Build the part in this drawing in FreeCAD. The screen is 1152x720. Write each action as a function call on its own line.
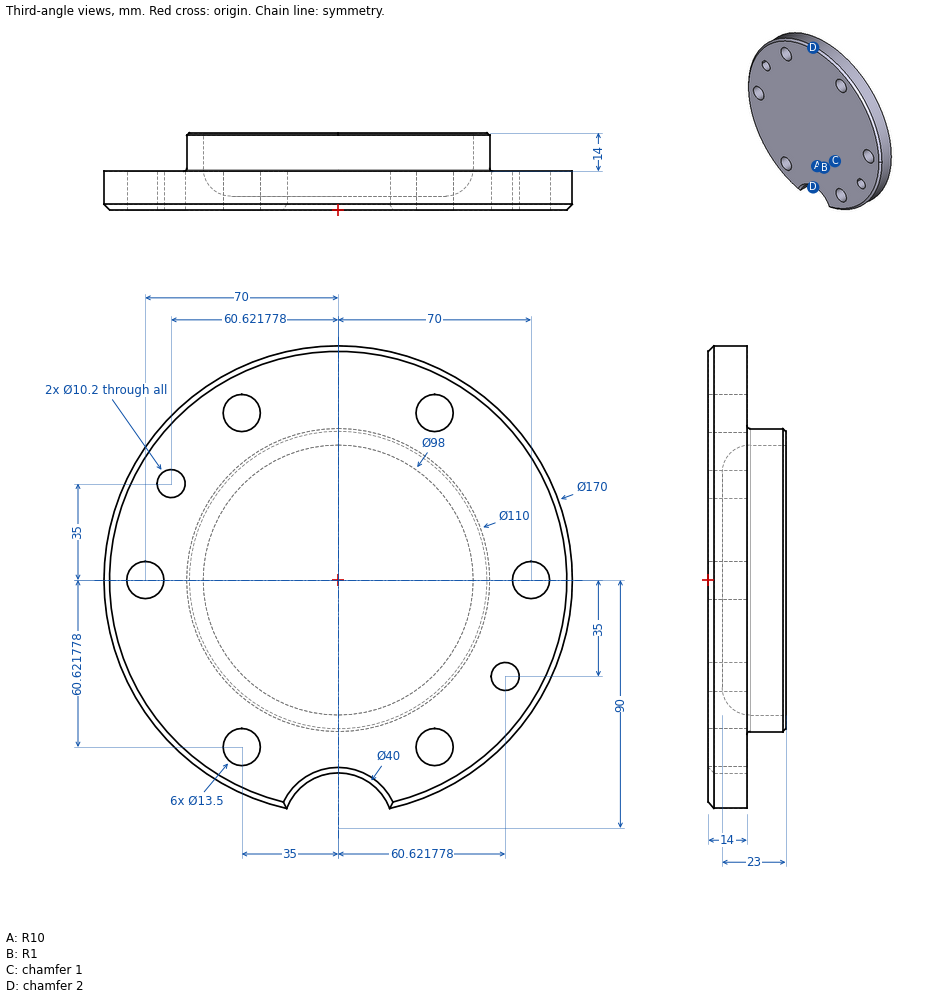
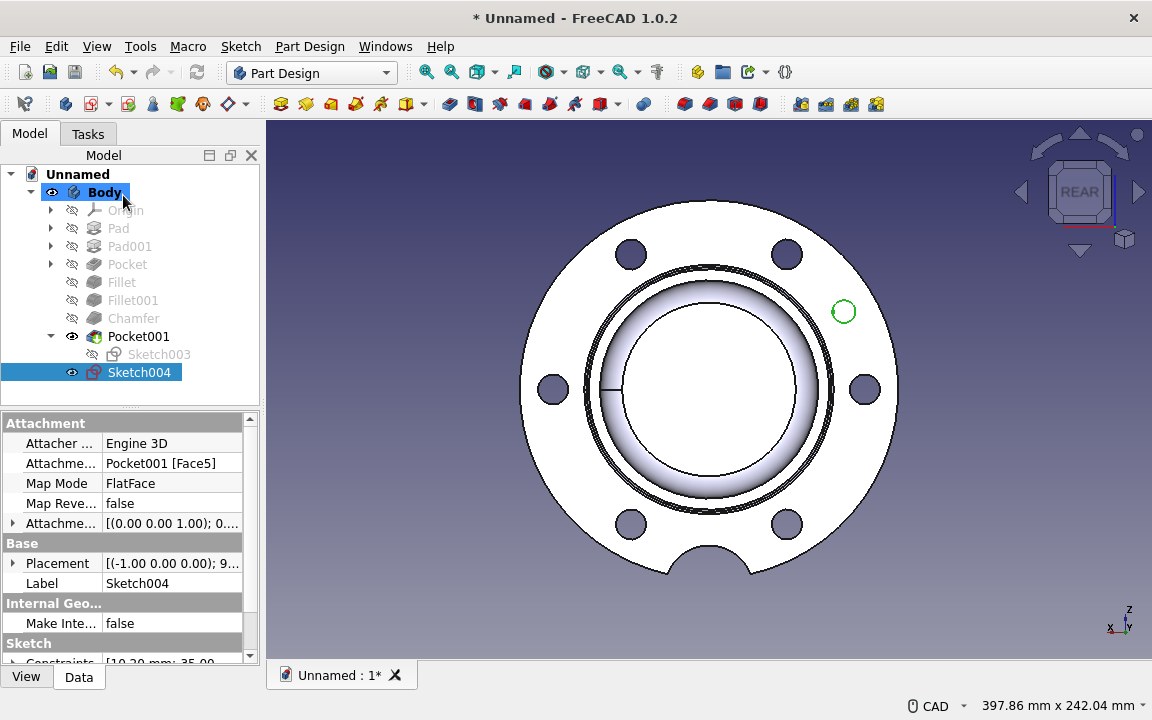
click(475, 104)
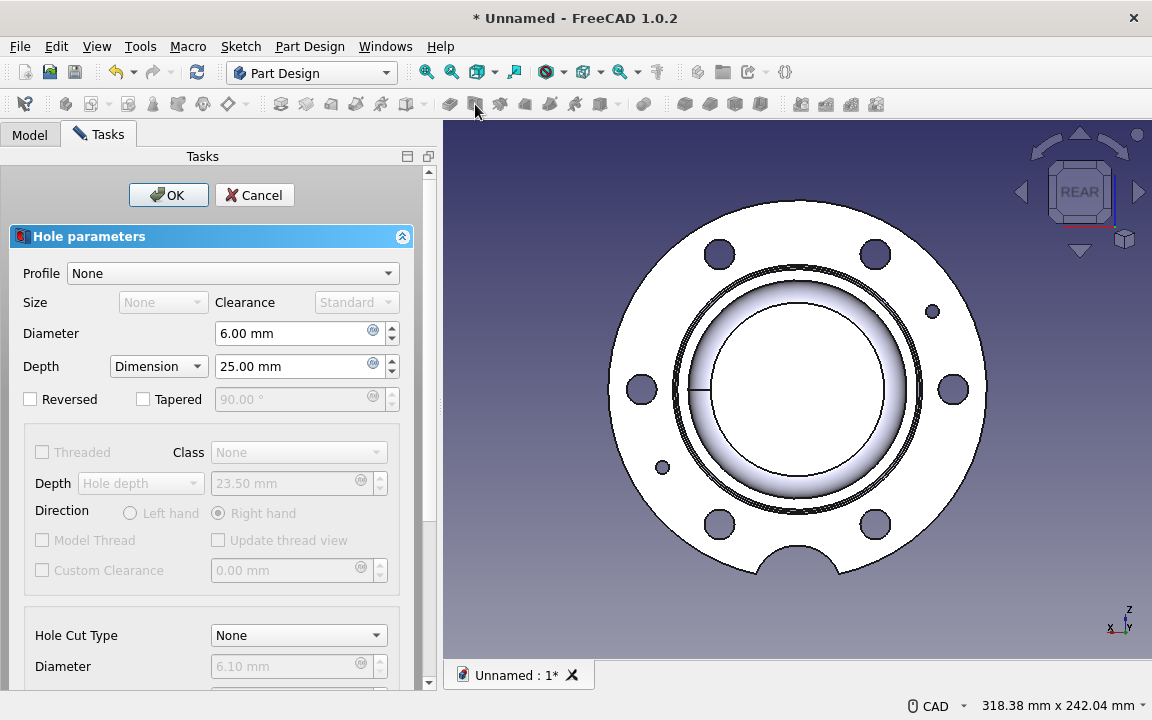
triple_click(300, 334)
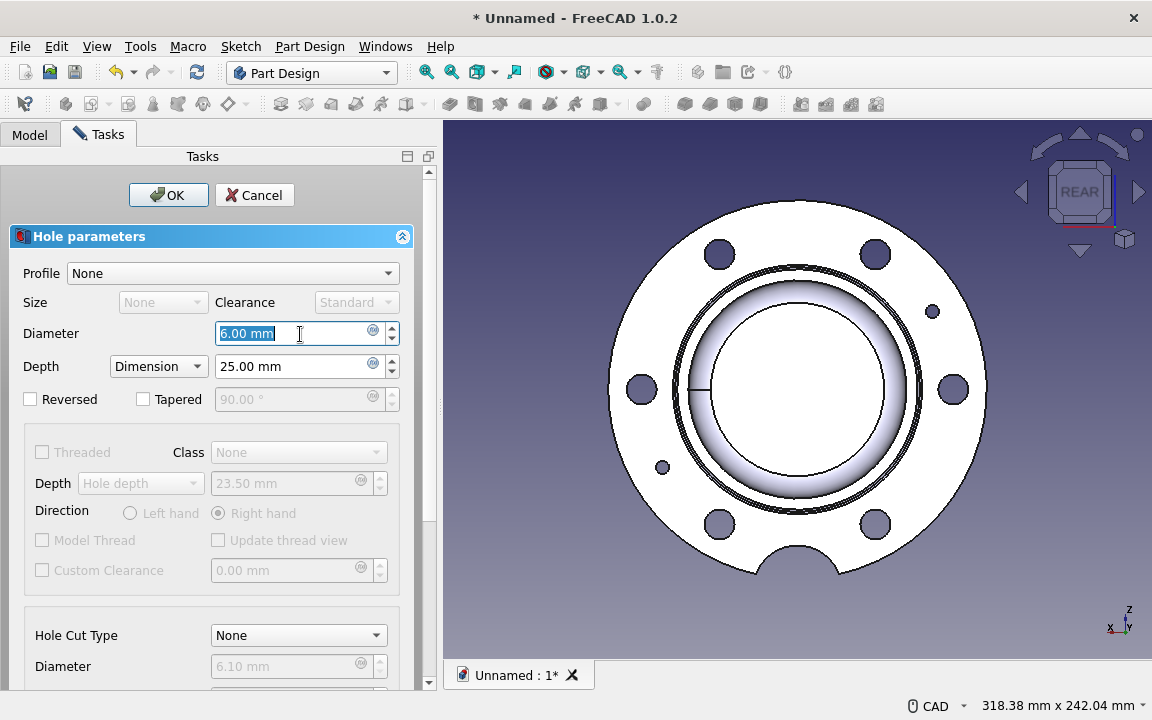
text(10.2)
key(Tab)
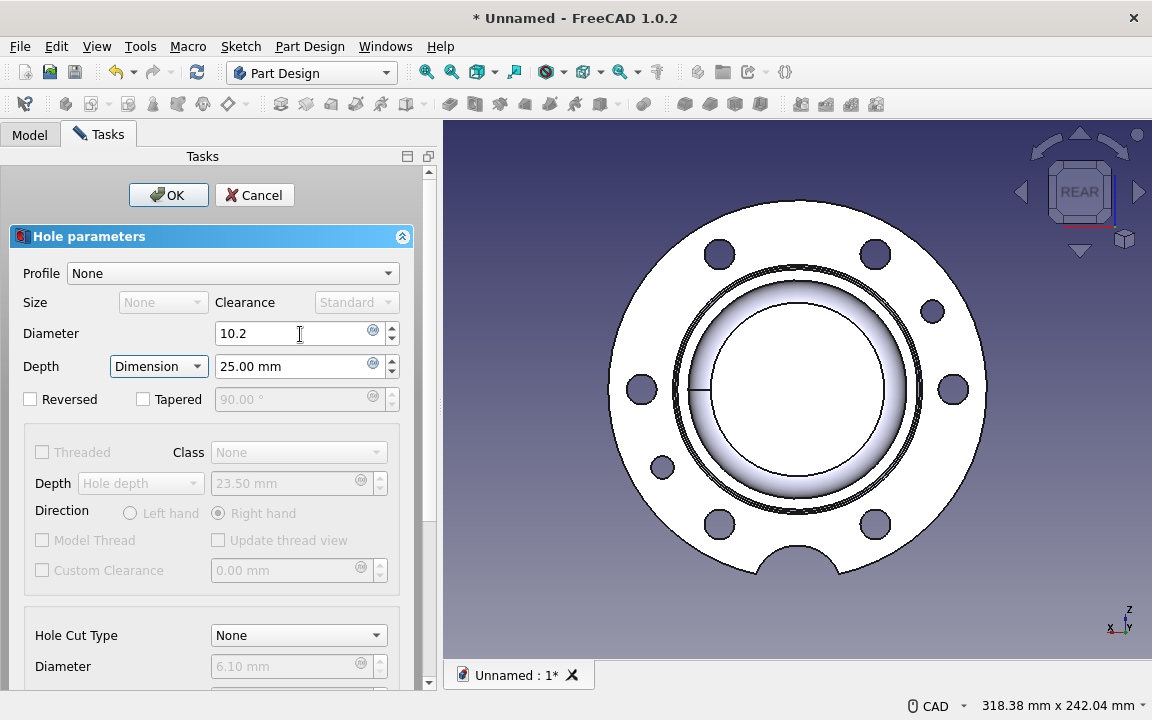
click(160, 366)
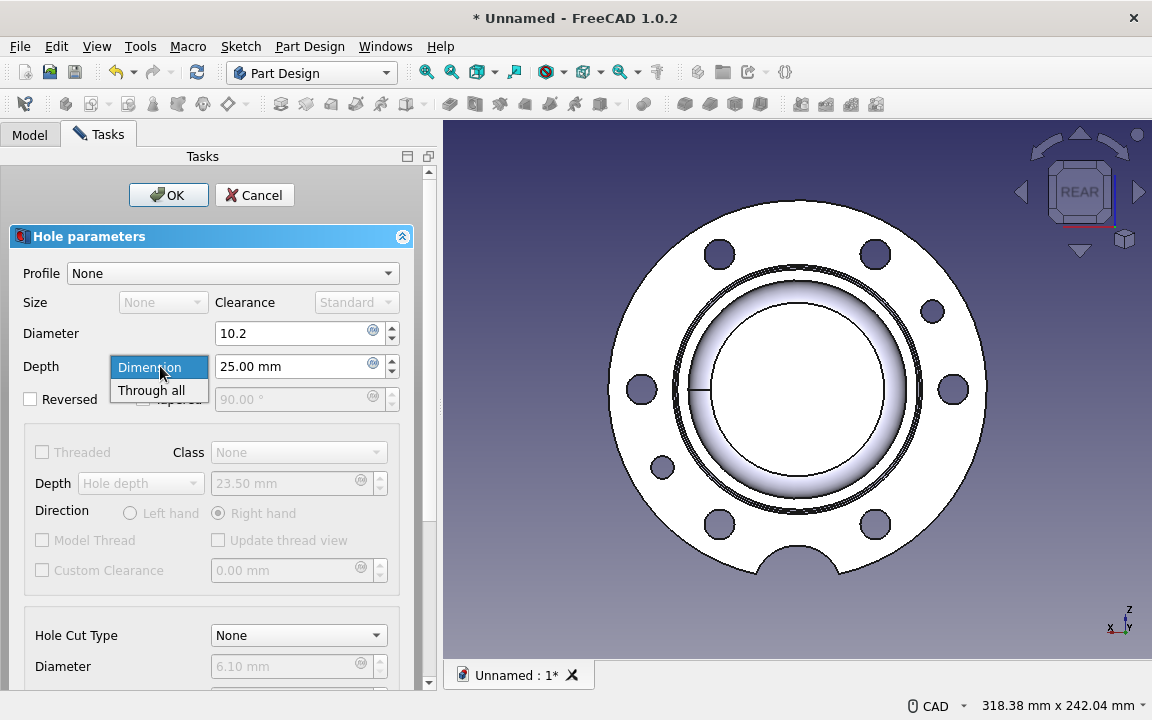
click(158, 390)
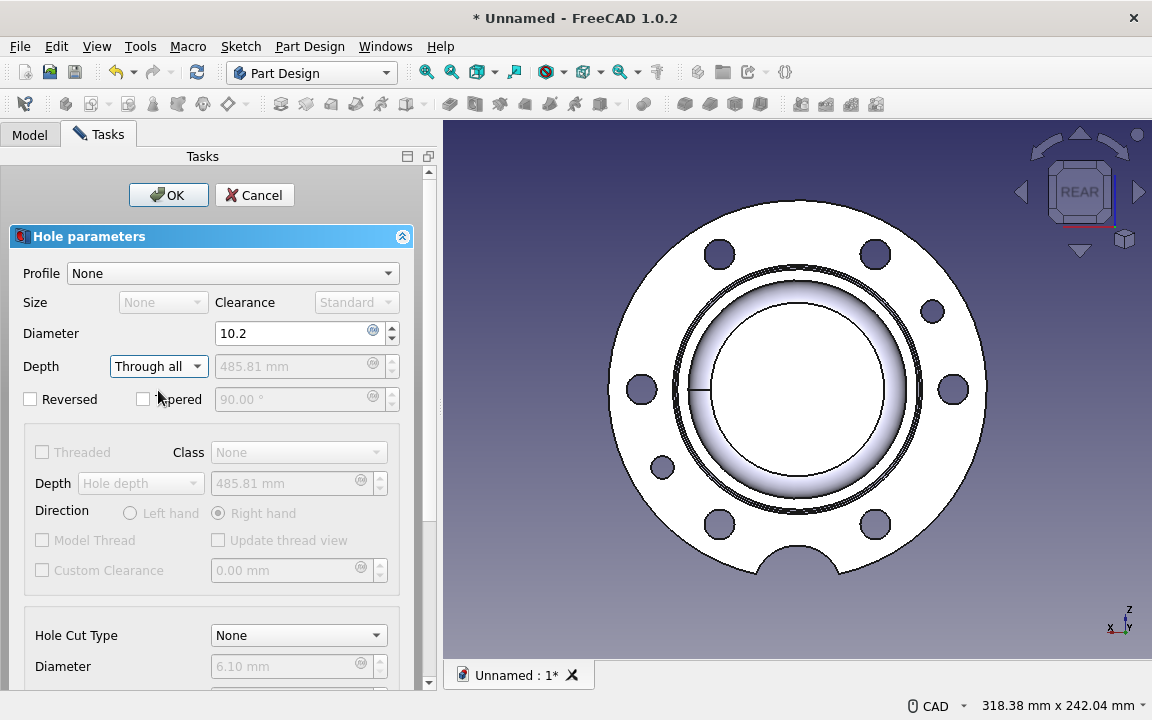
click(169, 195)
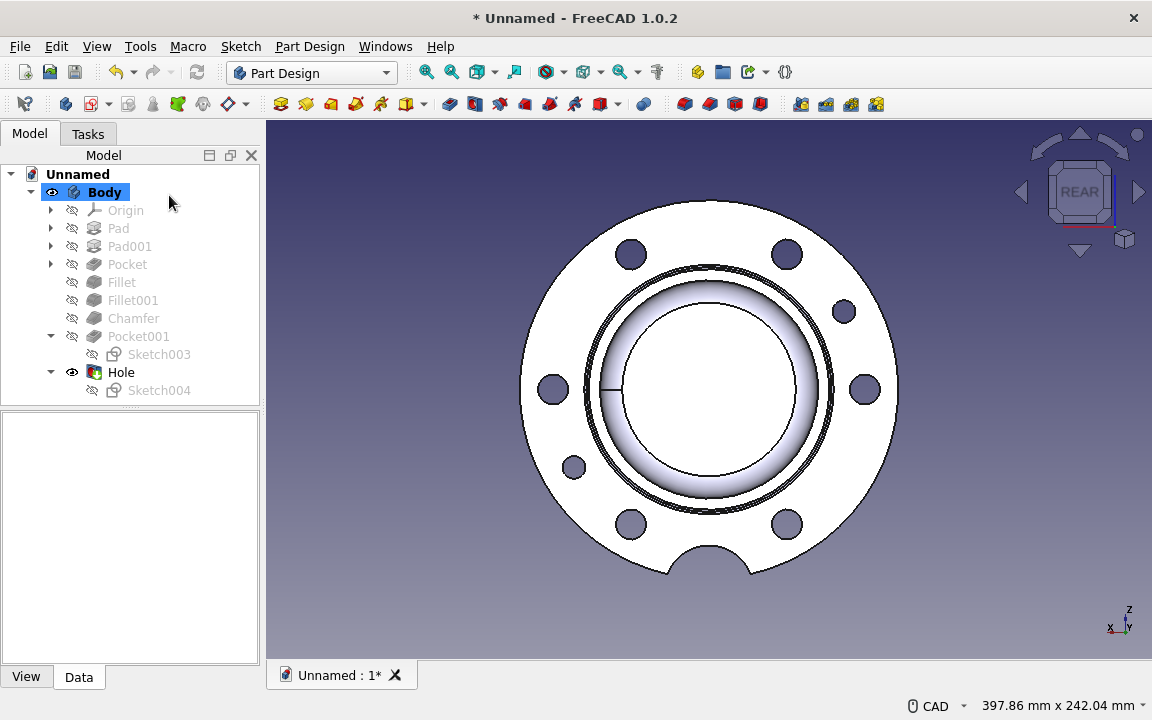
key(0)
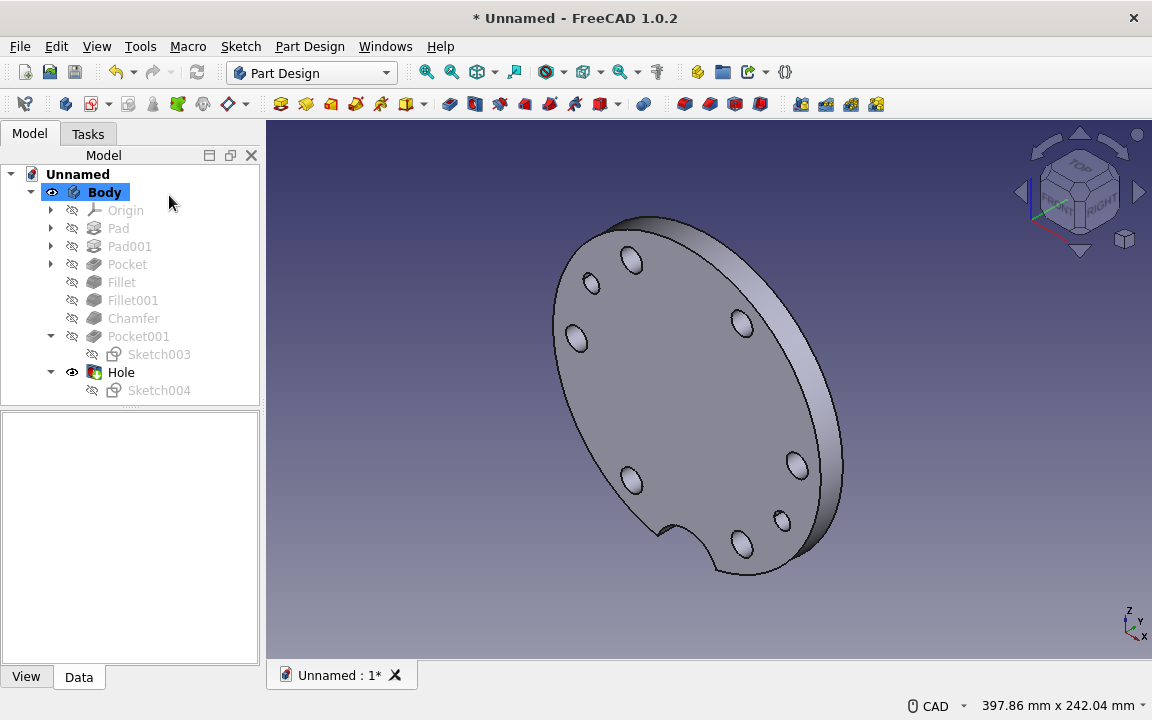
click(603, 232)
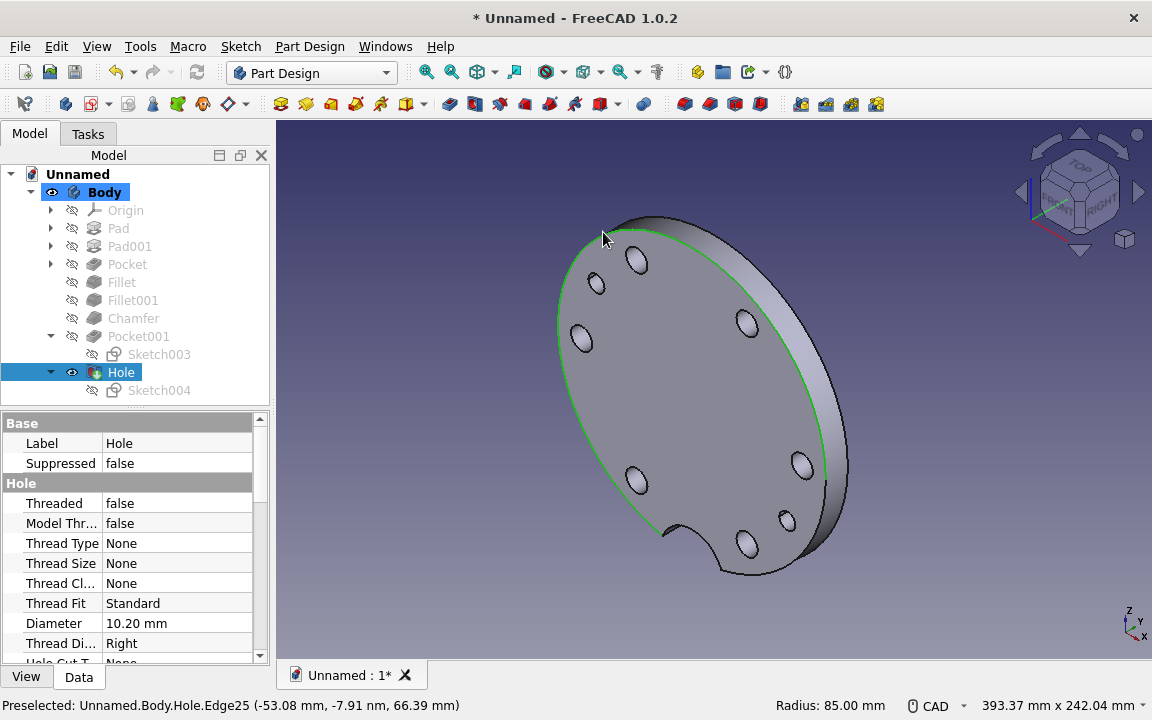
click(699, 534, ctrl)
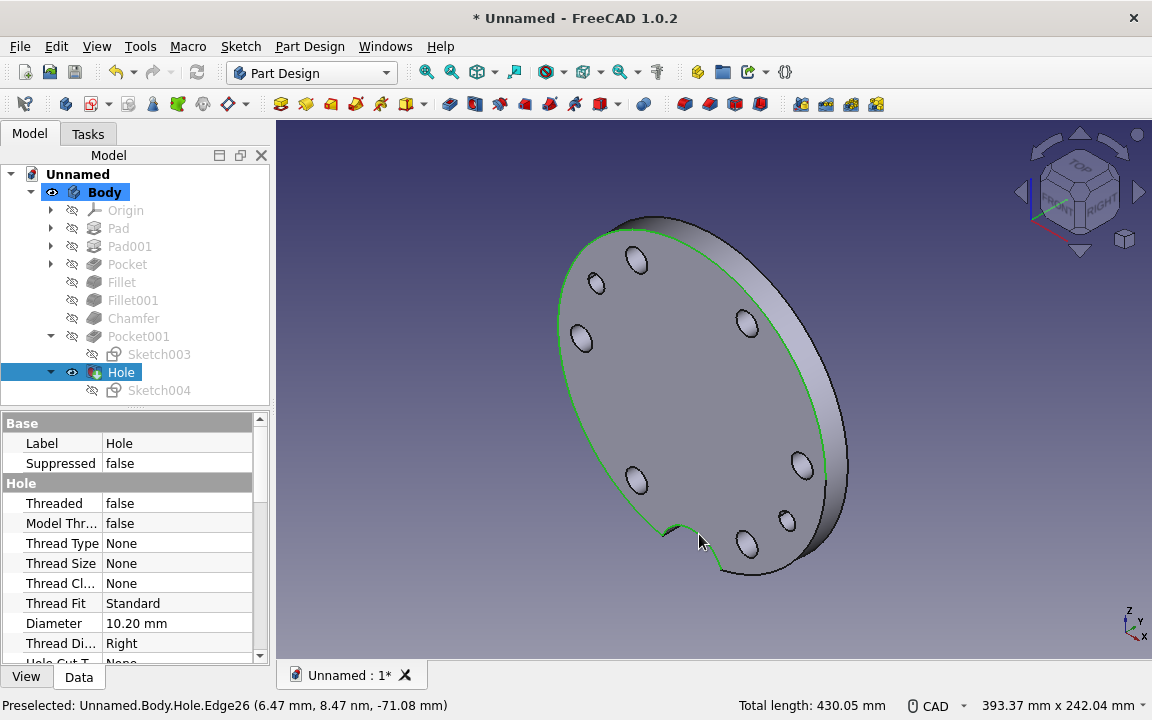
click(710, 104)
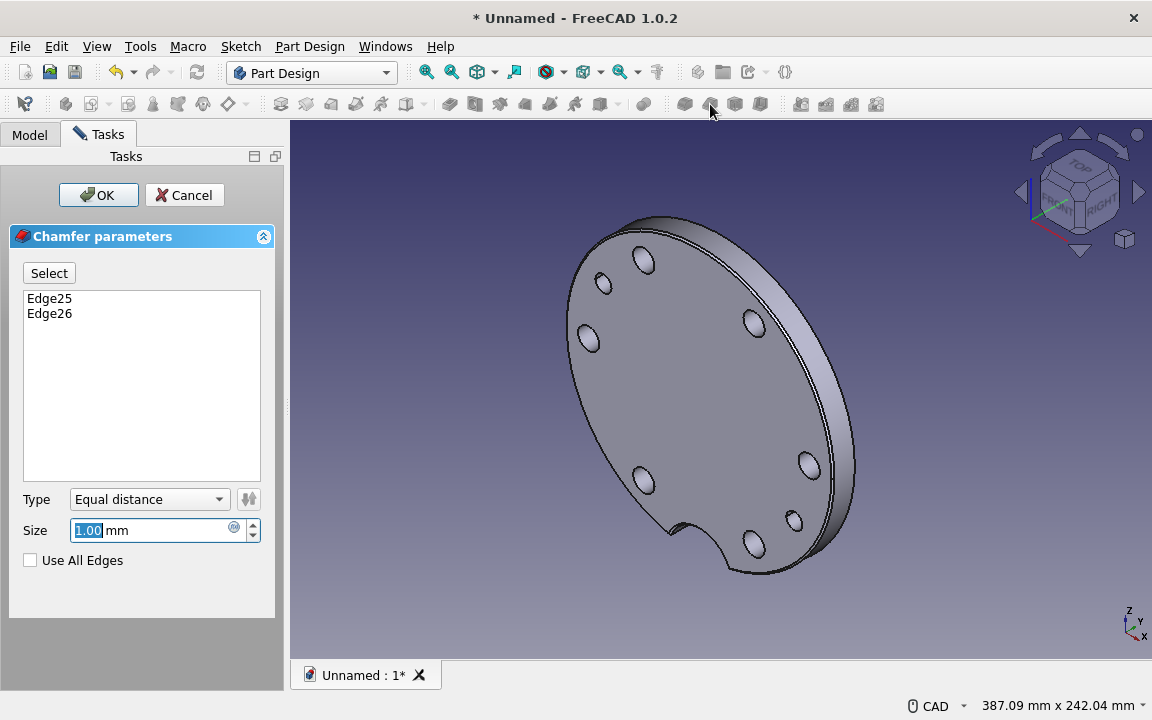
text(2)
key(Tab)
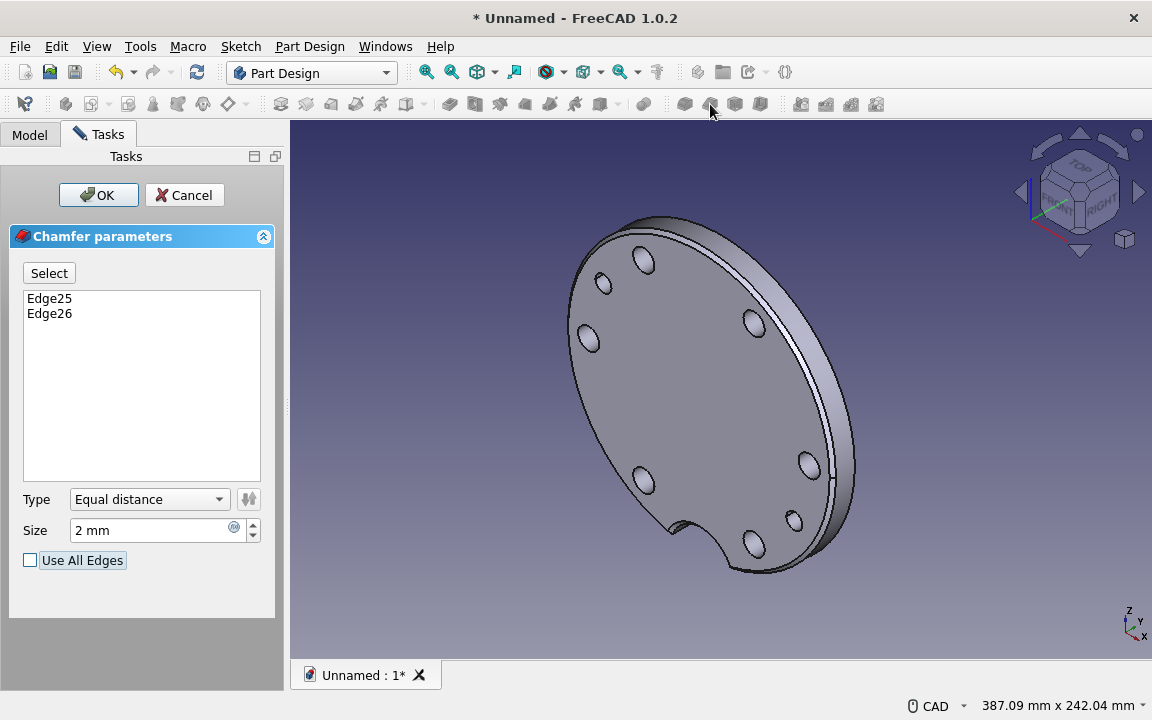
click(99, 195)